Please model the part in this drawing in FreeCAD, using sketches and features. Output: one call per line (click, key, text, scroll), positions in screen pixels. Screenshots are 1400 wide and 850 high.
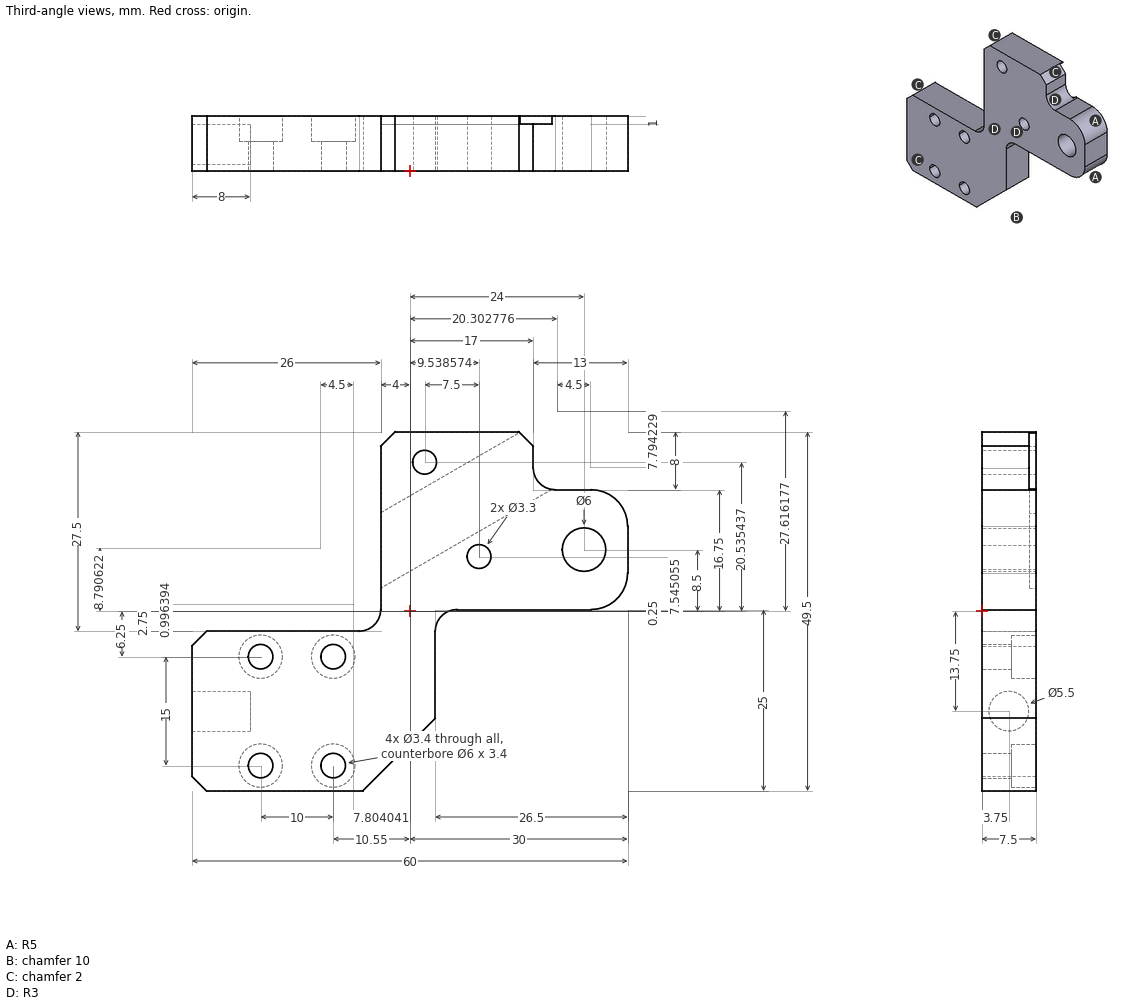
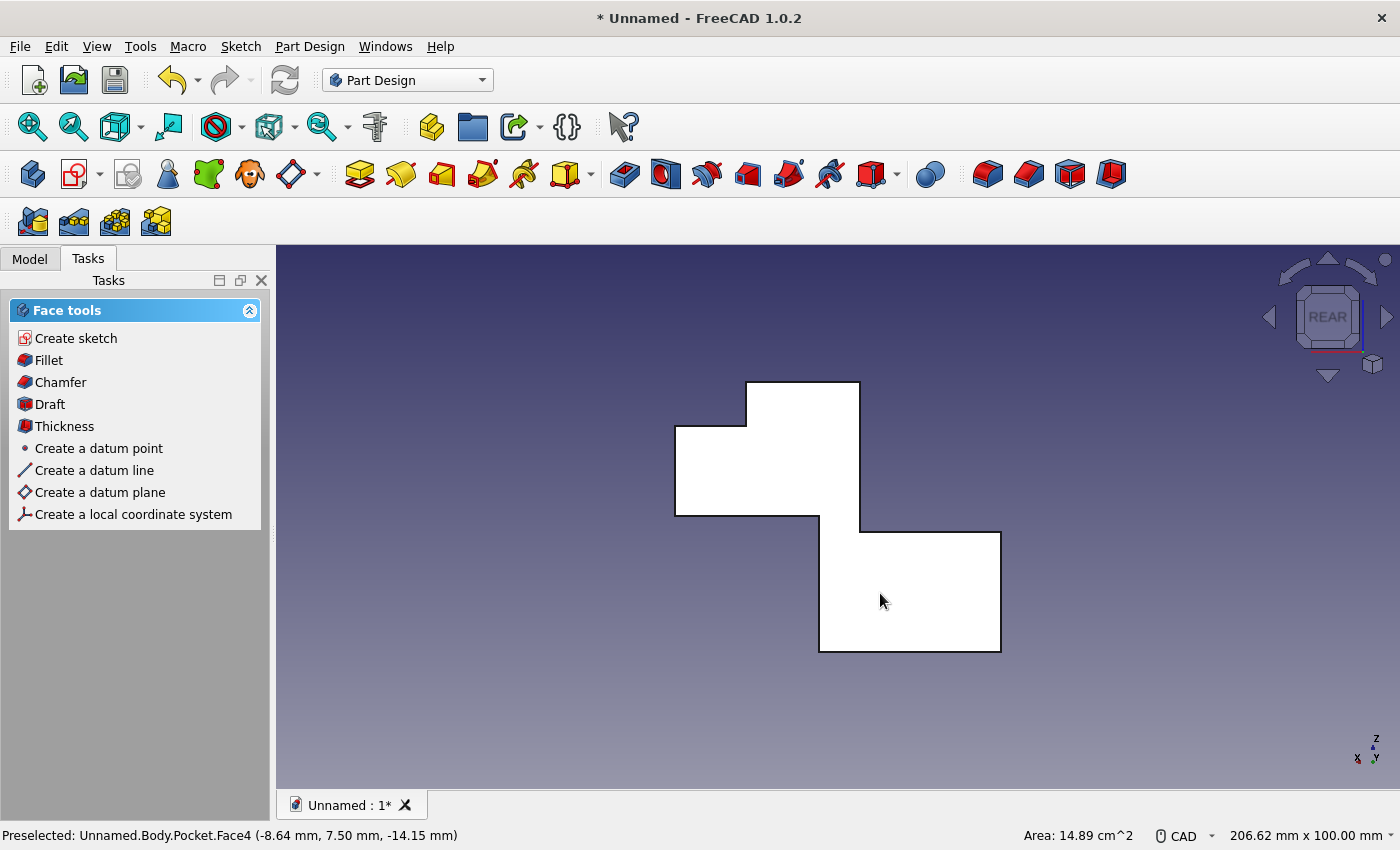
click(74, 174)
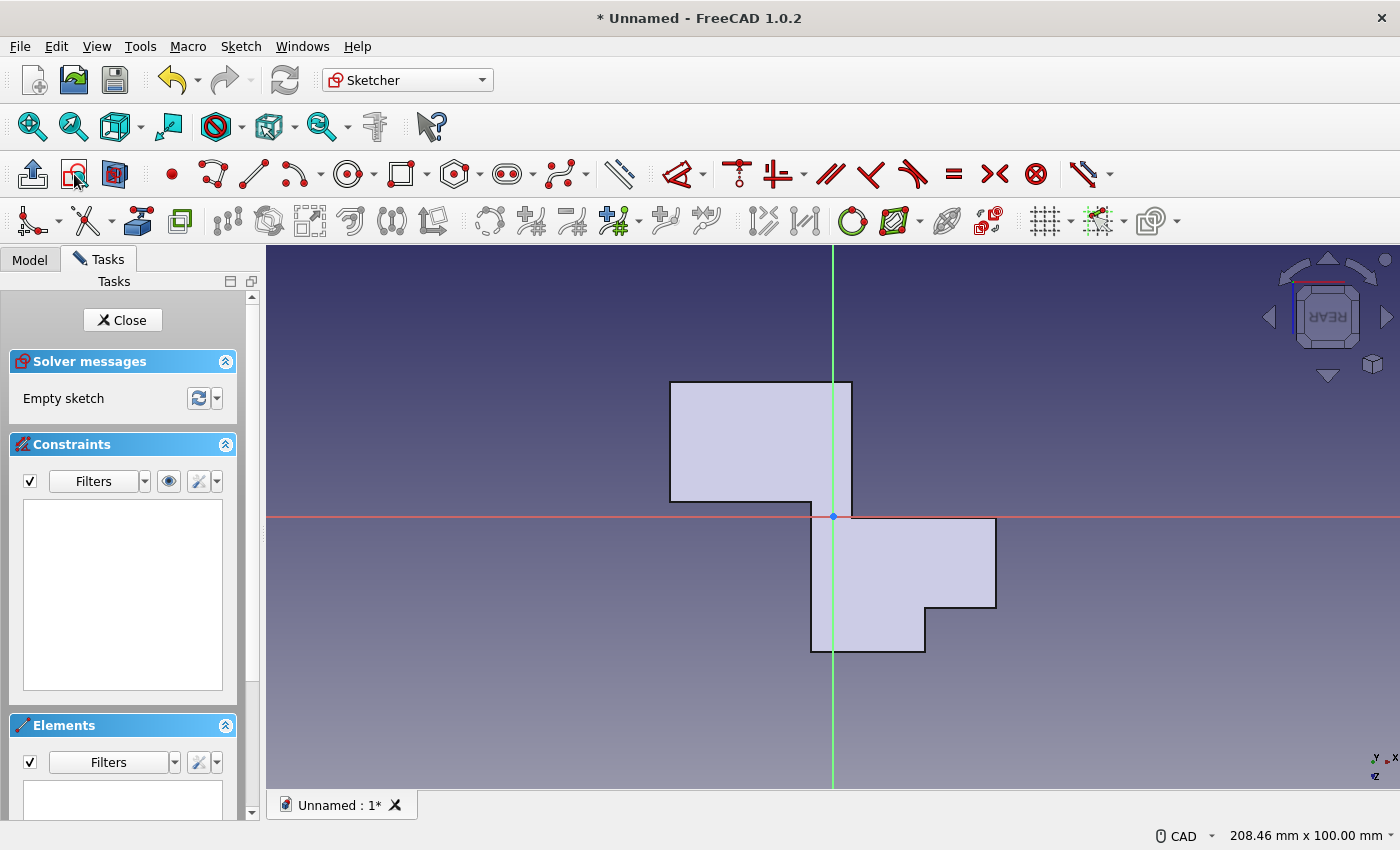
scroll(777, 418, up, 5)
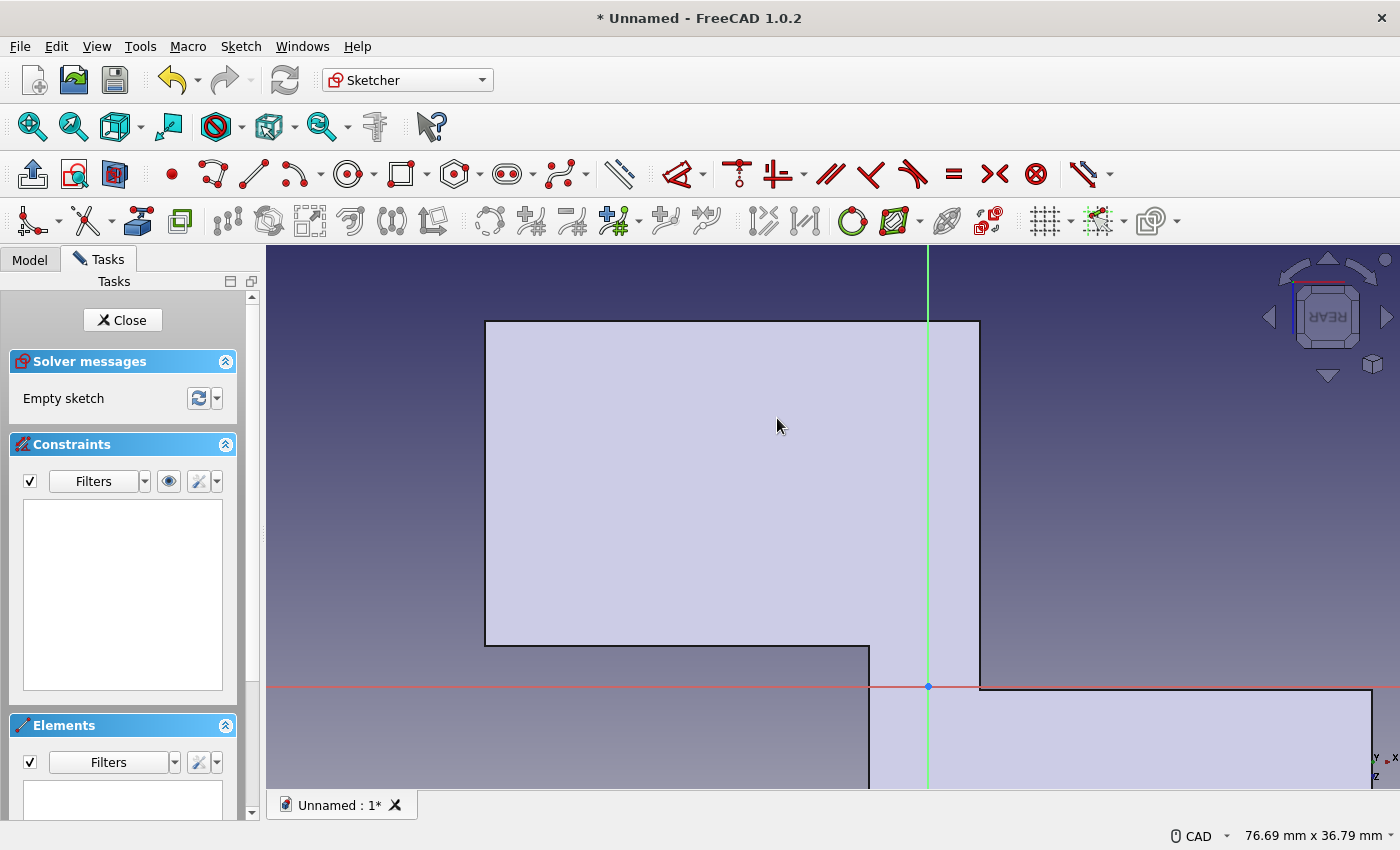
key(g)
key(c)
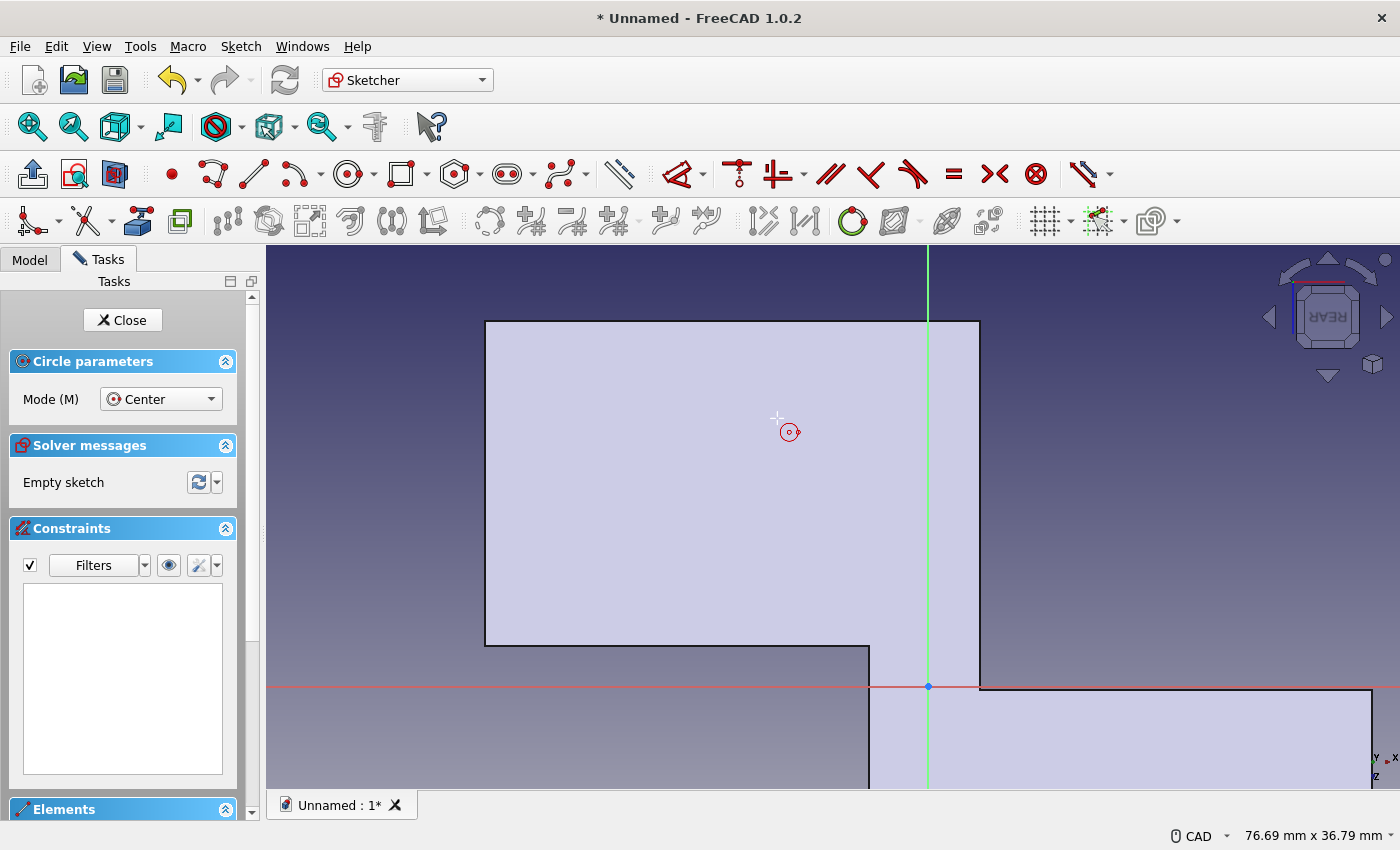
click(772, 372)
move(790, 355)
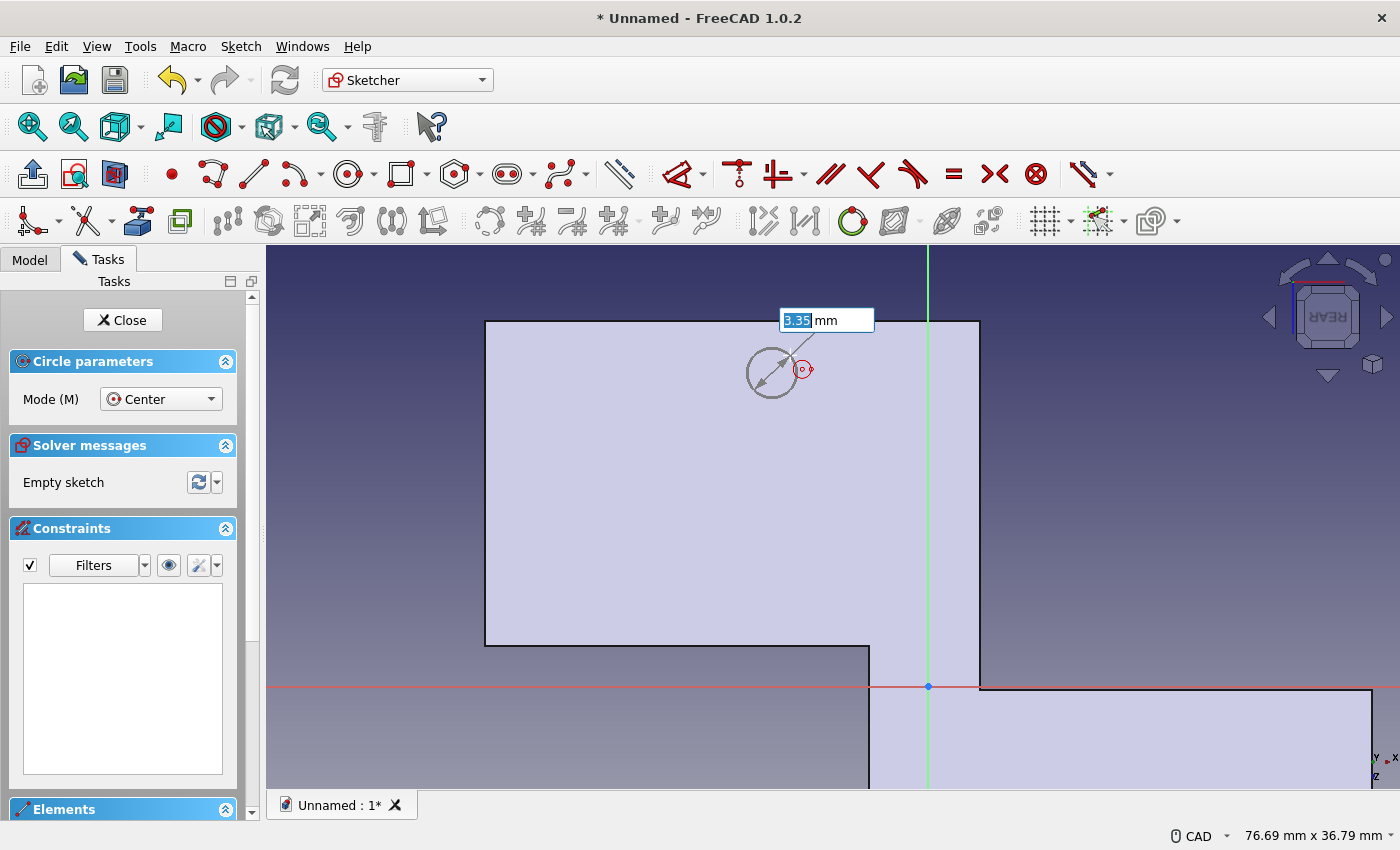
text(3.4)
key(Return)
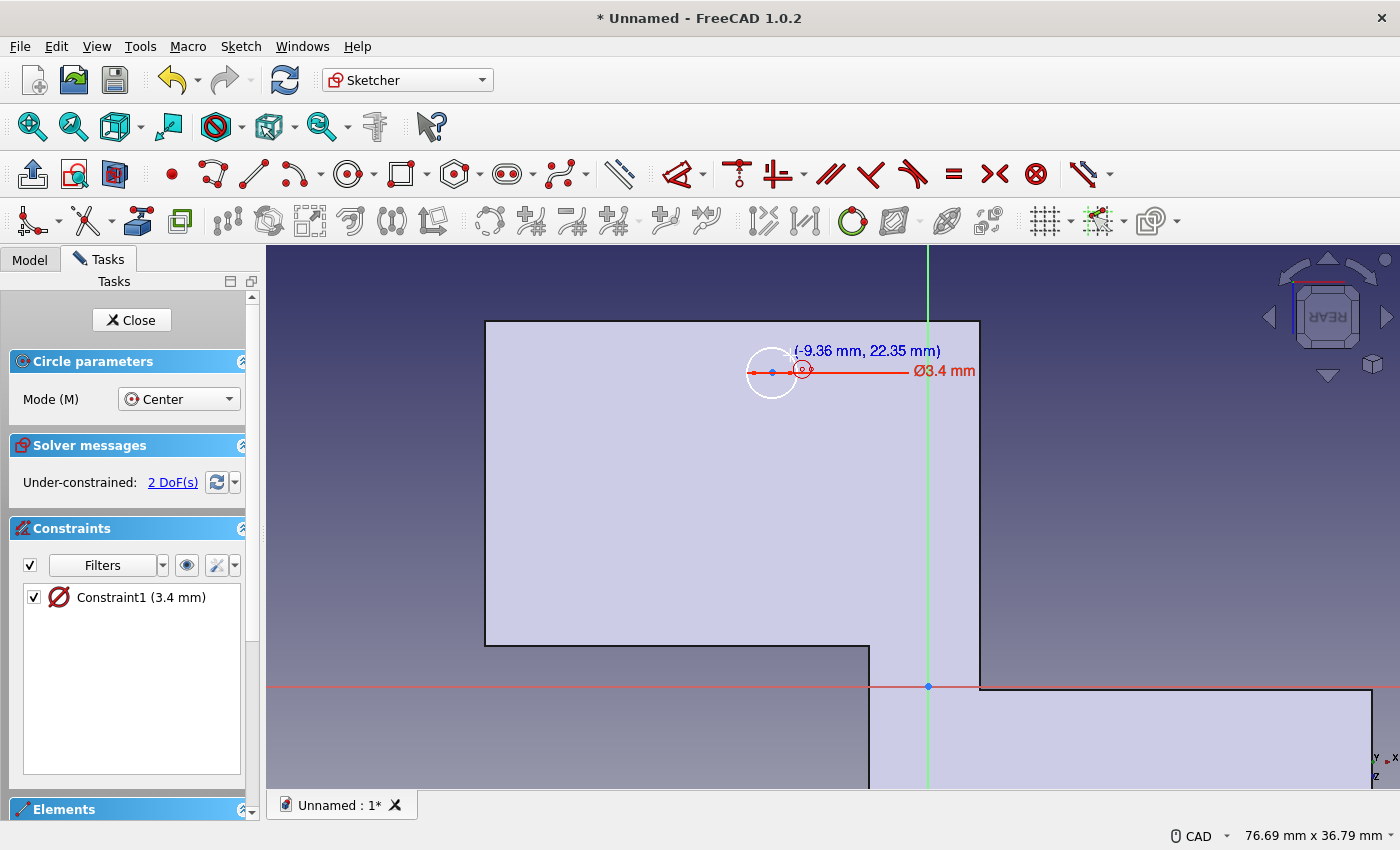
click(625, 372)
move(642, 355)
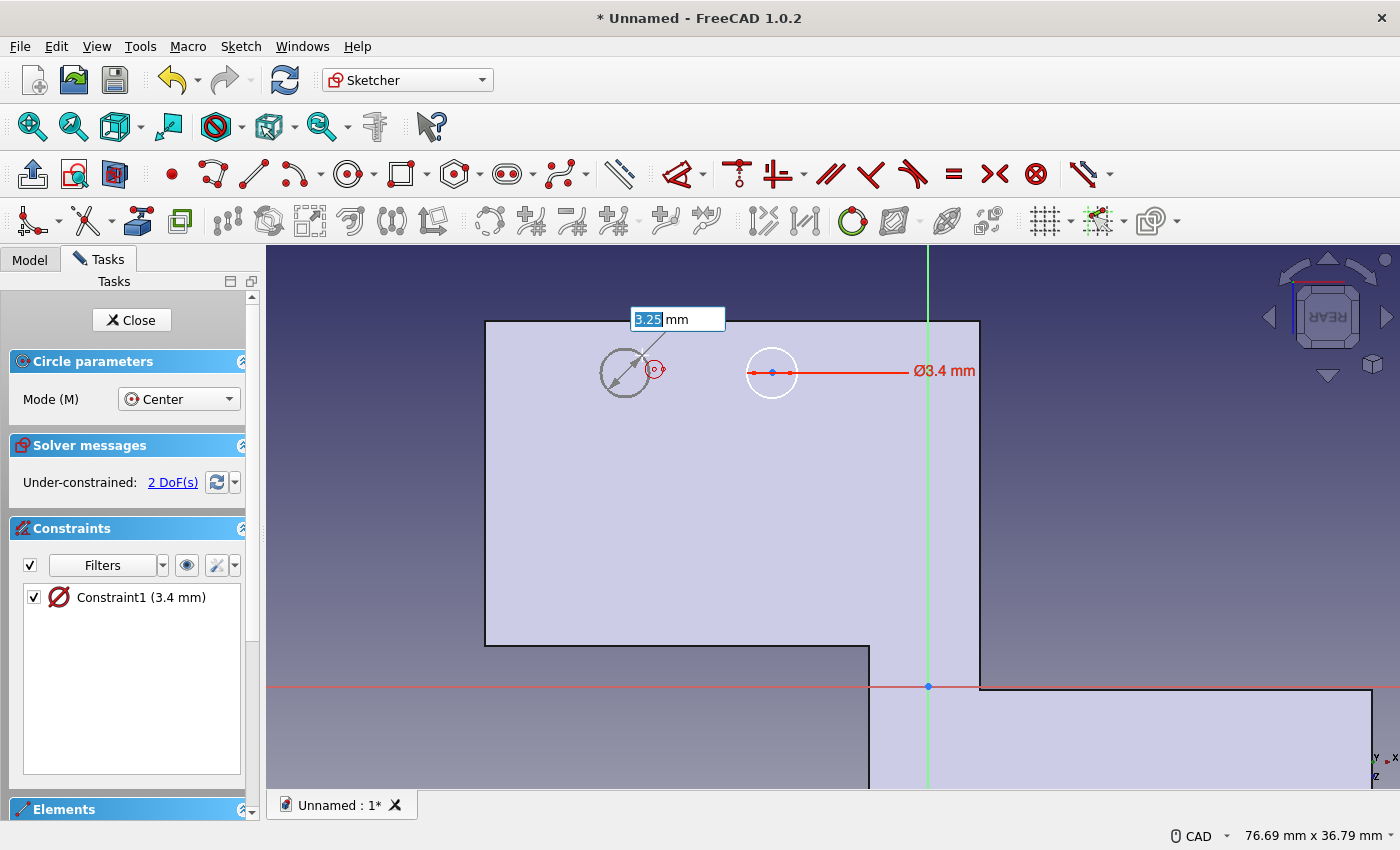
text(3.4)
key(Return)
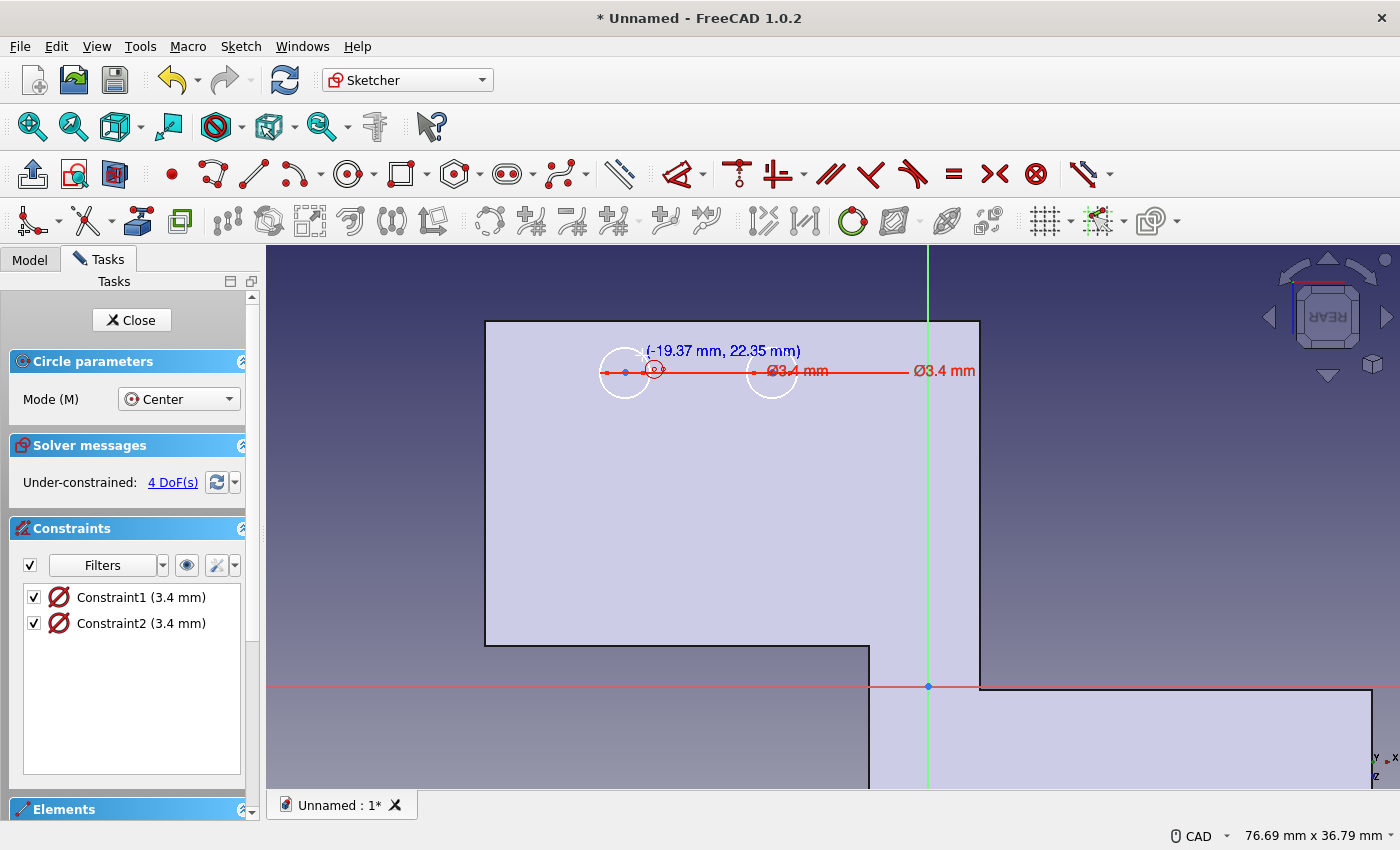
click(625, 594)
move(642, 576)